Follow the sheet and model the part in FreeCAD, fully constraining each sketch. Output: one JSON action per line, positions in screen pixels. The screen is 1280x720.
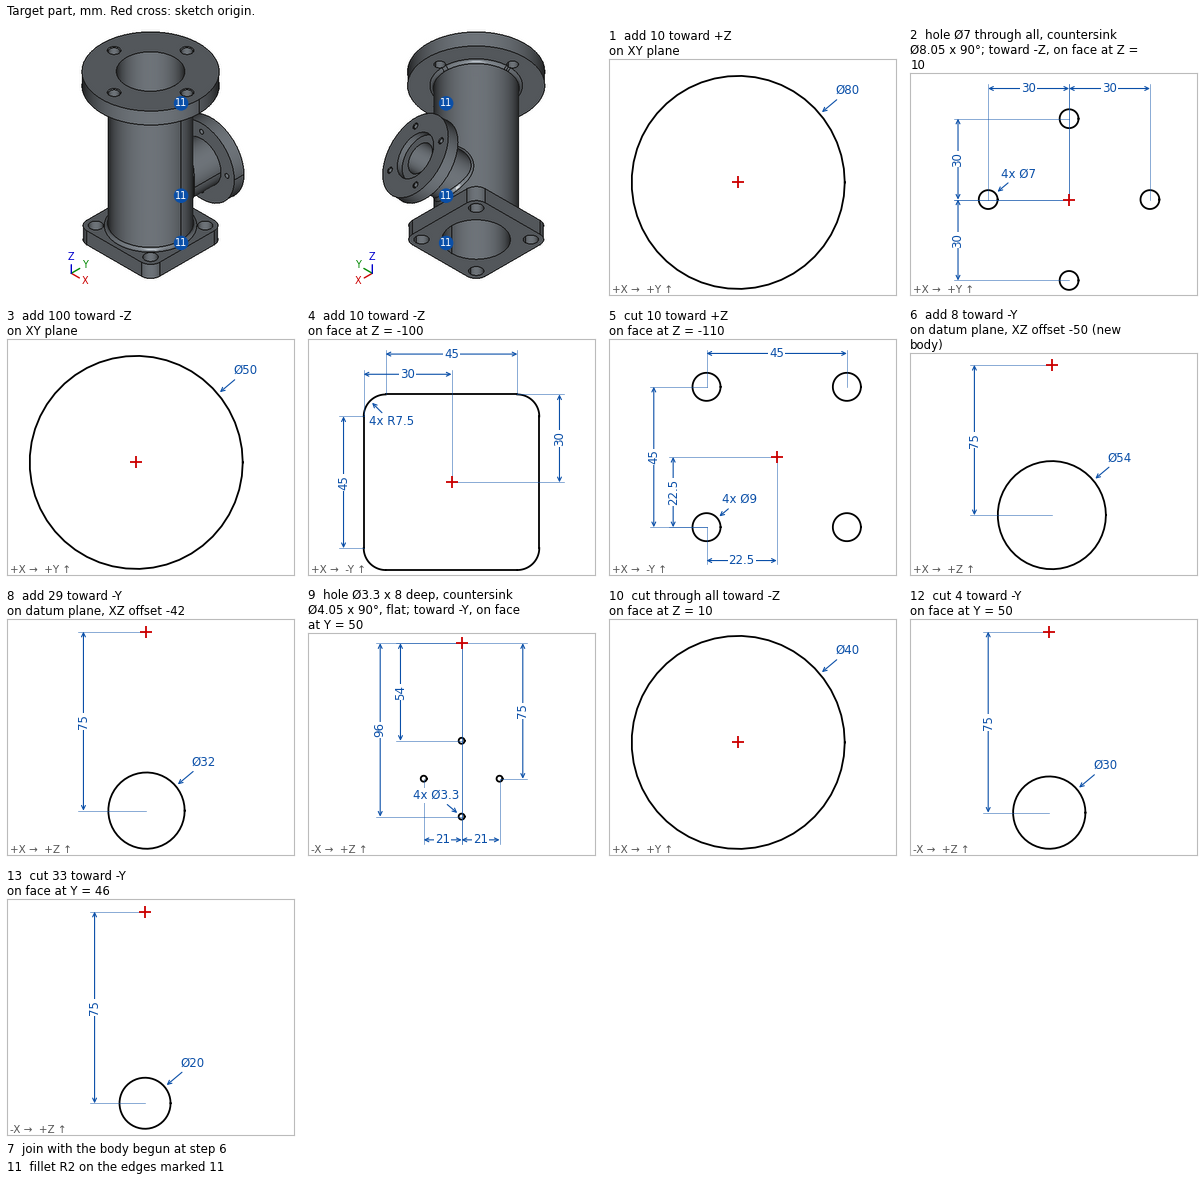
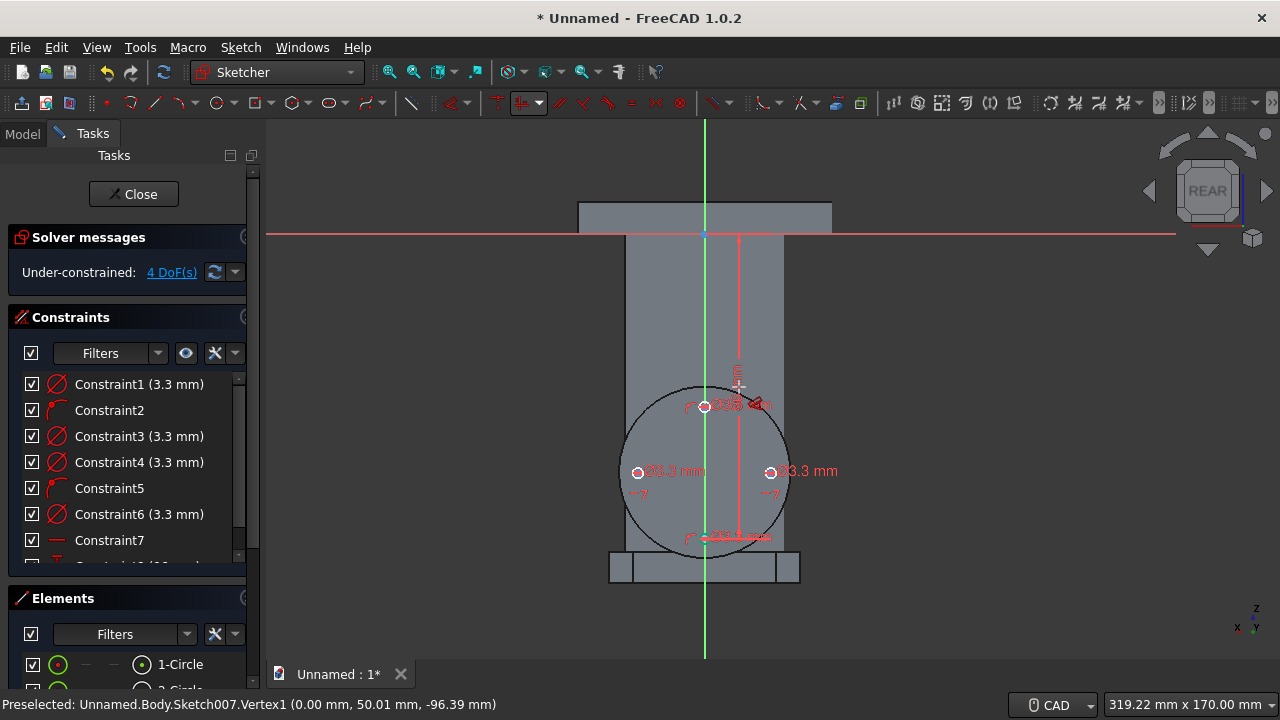
{"action": "left_click", "coordinate": [771, 473]}
{"action": "left_click", "coordinate": [738, 200]}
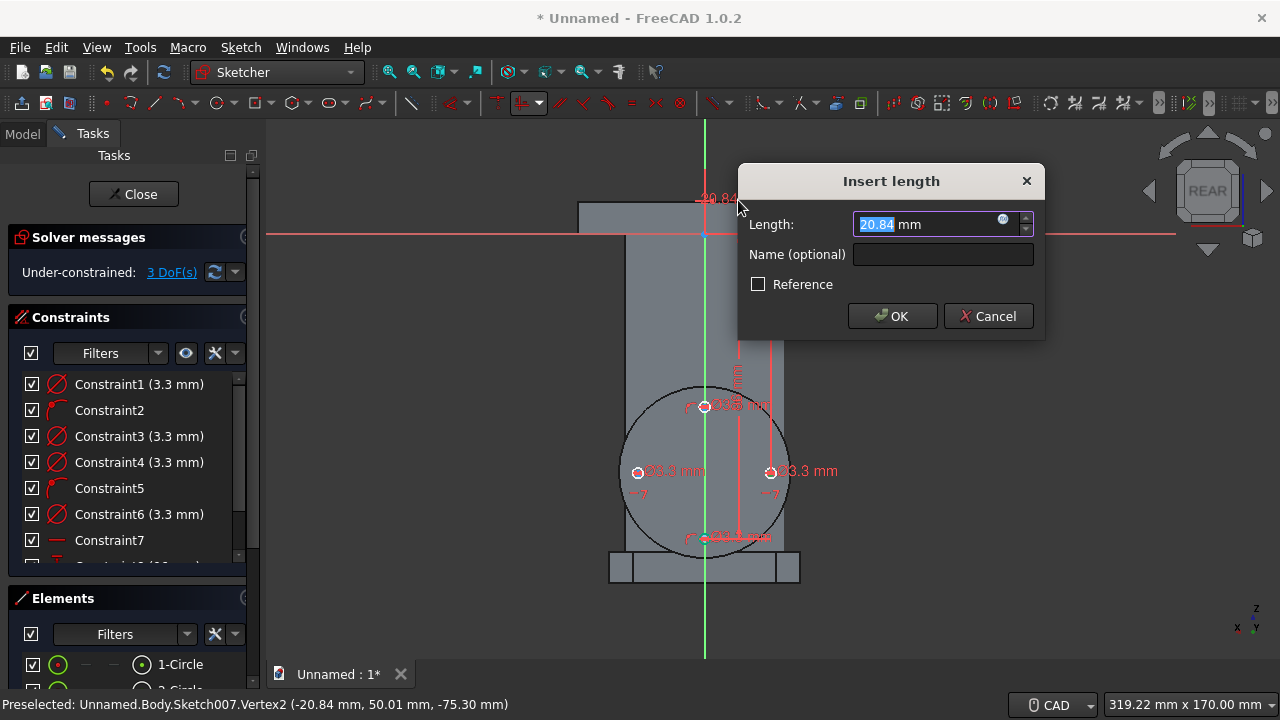
{"action": "type", "text": "21"}
{"action": "key", "text": "Return"}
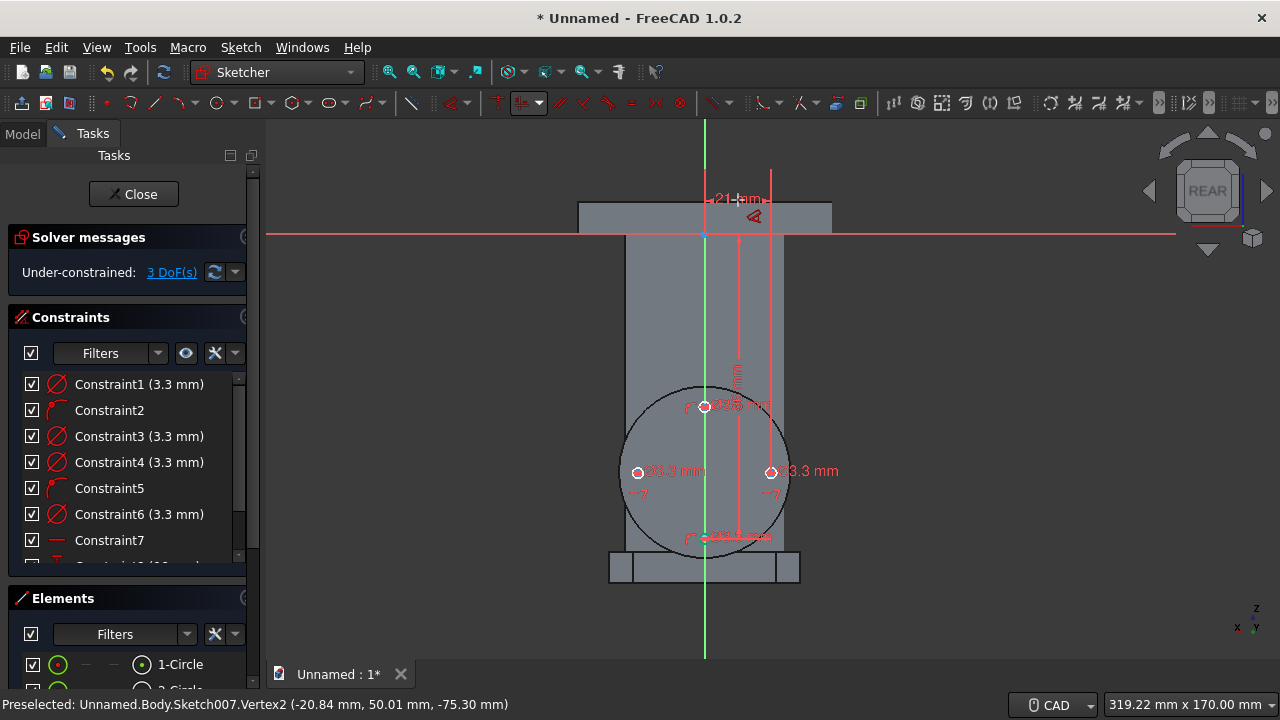
{"action": "left_click", "coordinate": [771, 473]}
{"action": "left_click", "coordinate": [805, 354]}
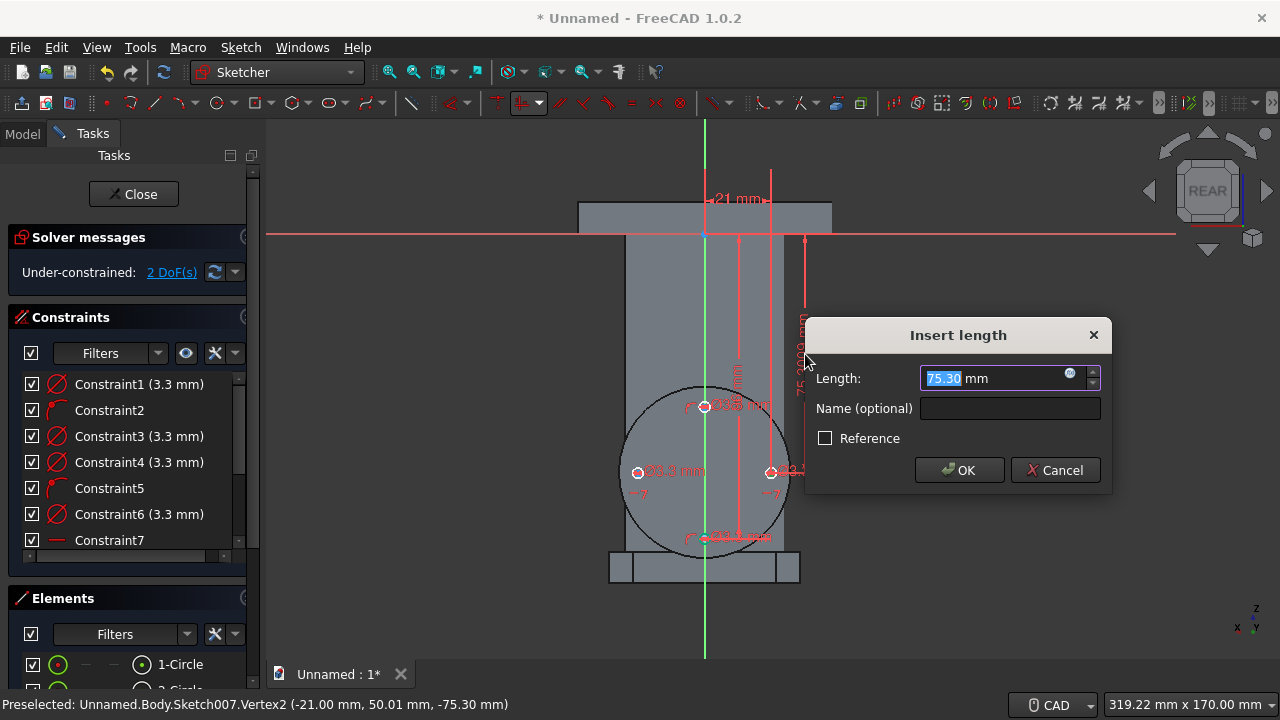
{"action": "type", "text": "75"}
{"action": "key", "text": "Return"}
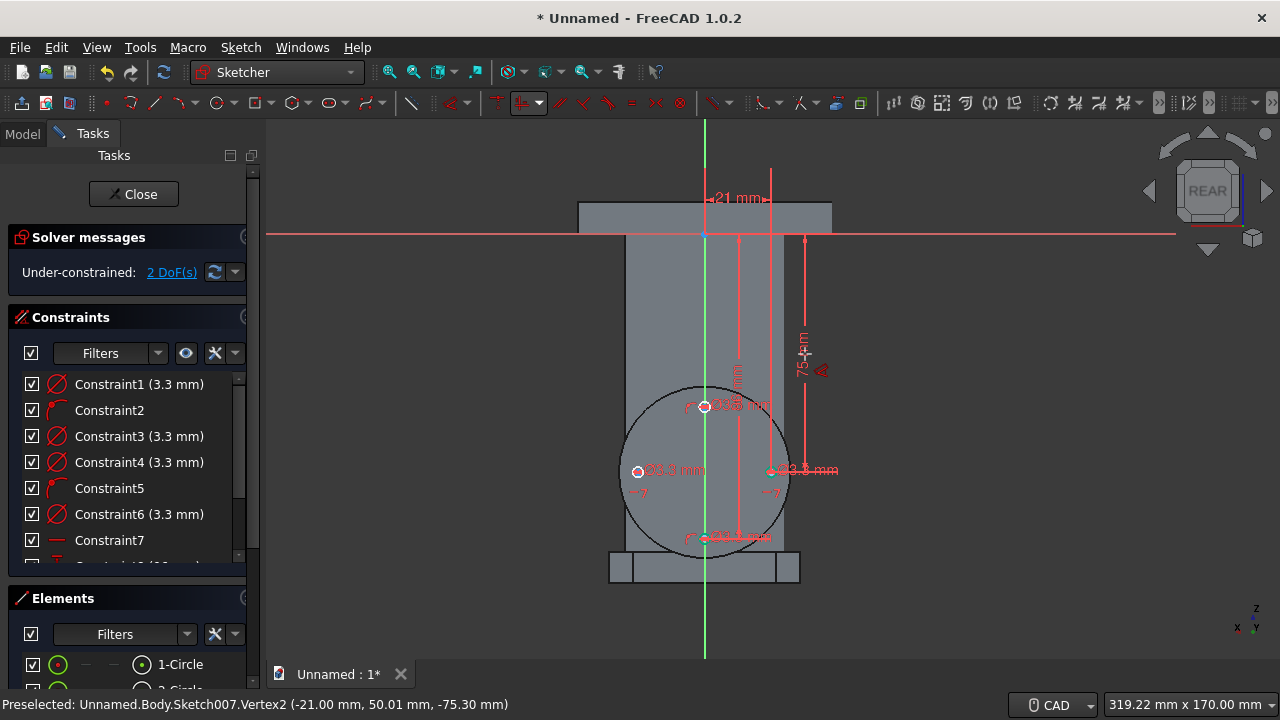
{"action": "left_click", "coordinate": [705, 407]}
{"action": "left_click", "coordinate": [739, 321]}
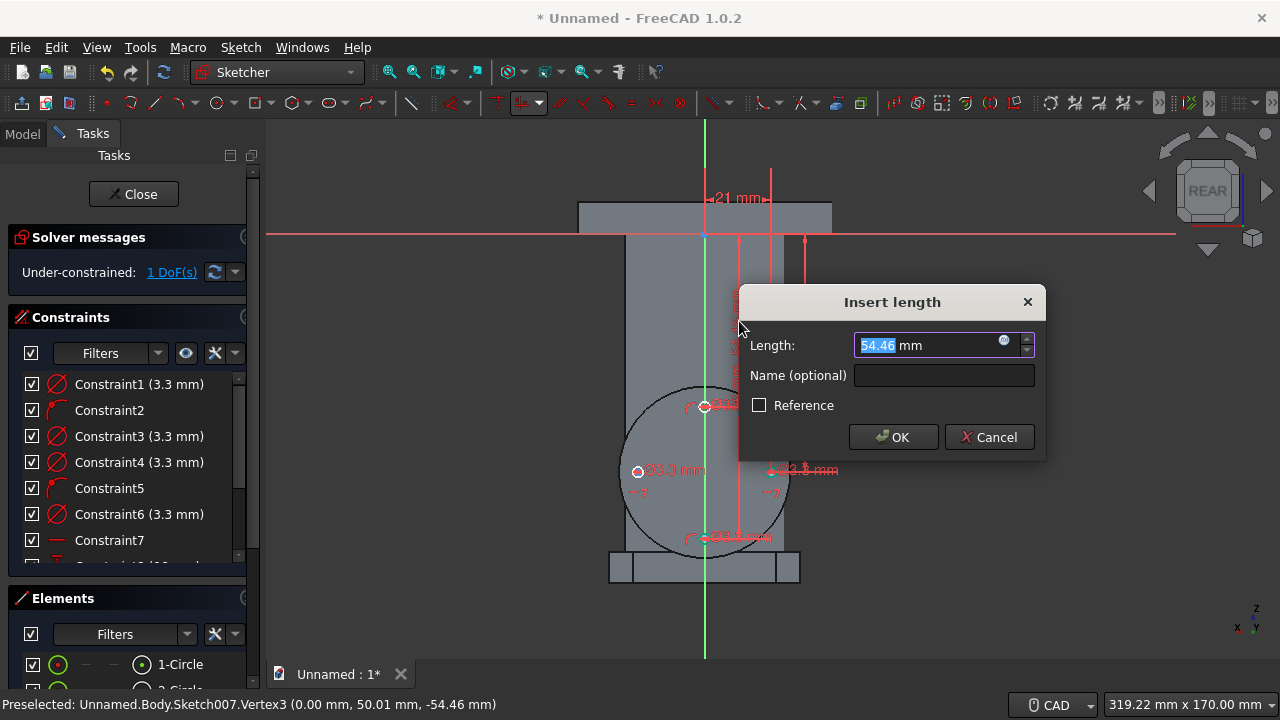
{"action": "type", "text": "54"}
{"action": "key", "text": "Return"}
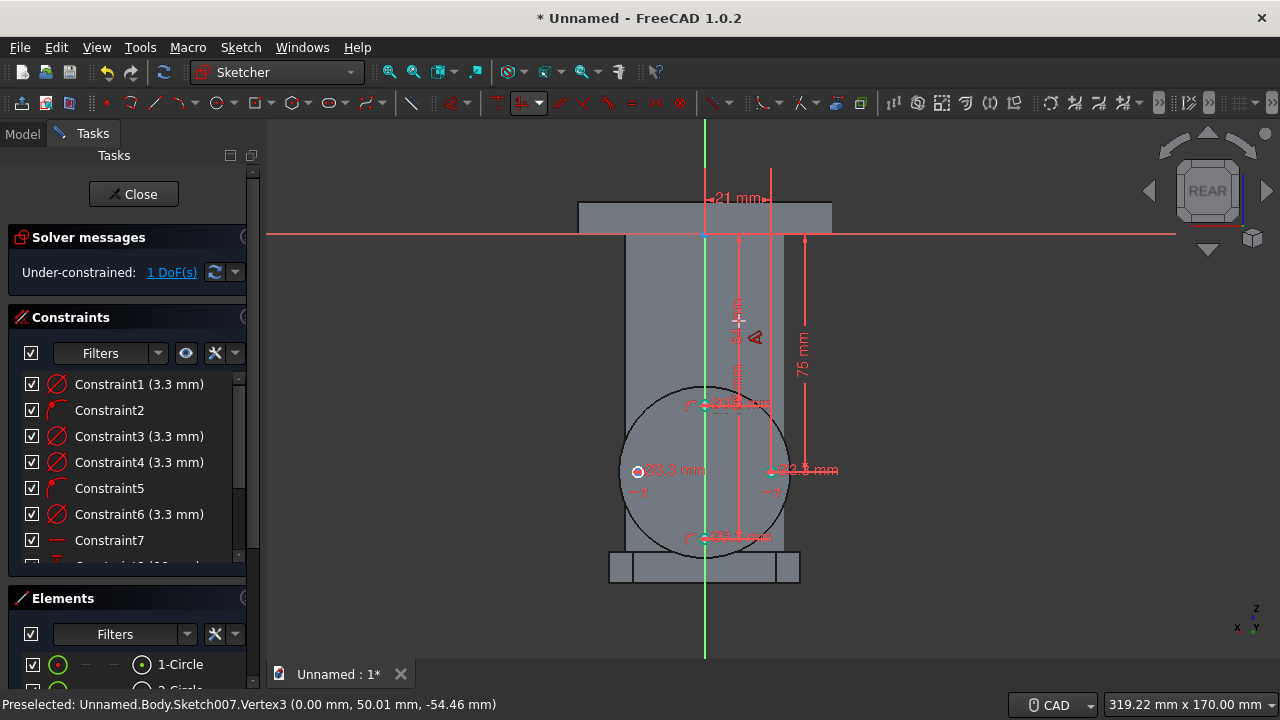
{"action": "left_click", "coordinate": [638, 472]}
{"action": "left_click", "coordinate": [656, 200]}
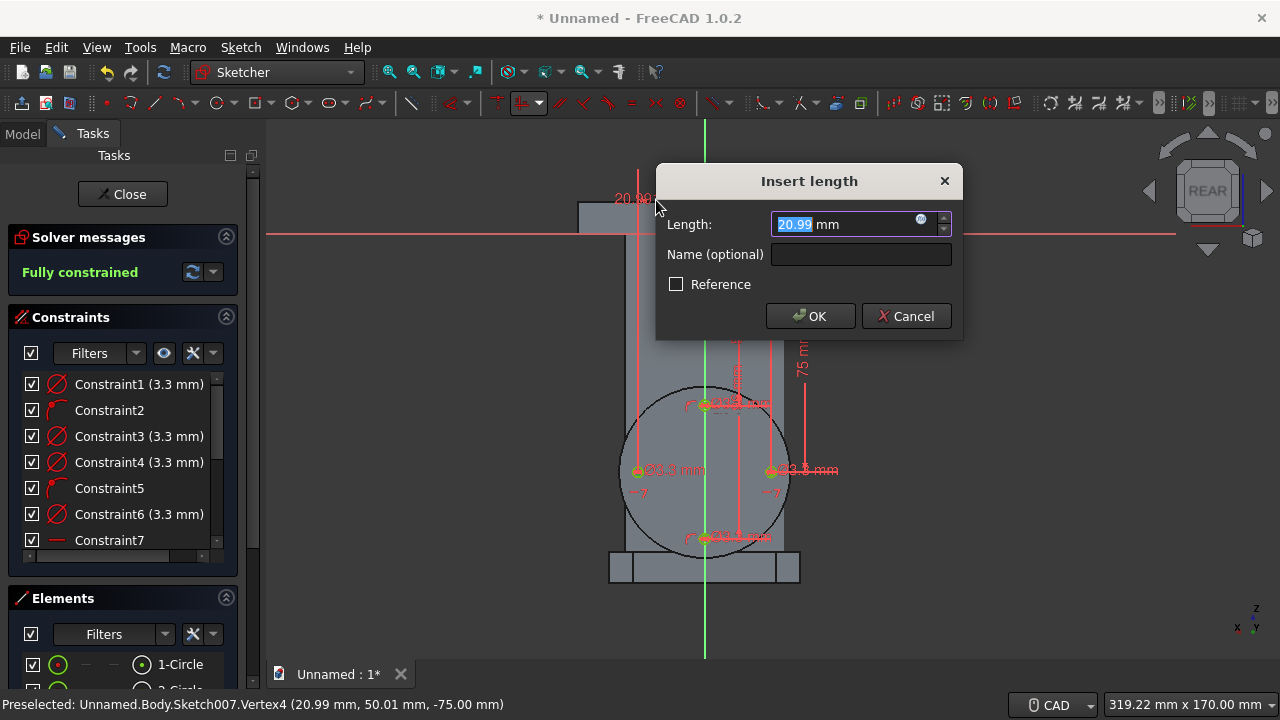
{"action": "type", "text": "21"}
{"action": "key", "text": "Return"}
{"action": "key", "text": "Escape"}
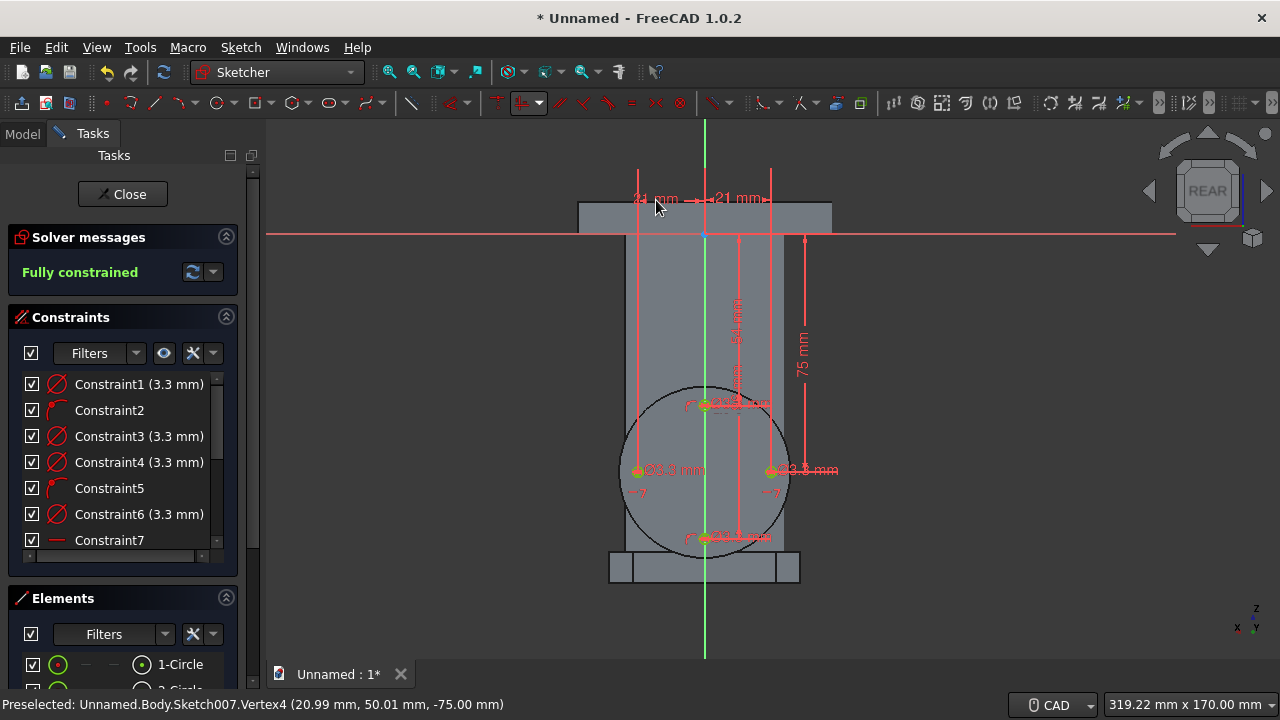
{"action": "left_click", "coordinate": [123, 194]}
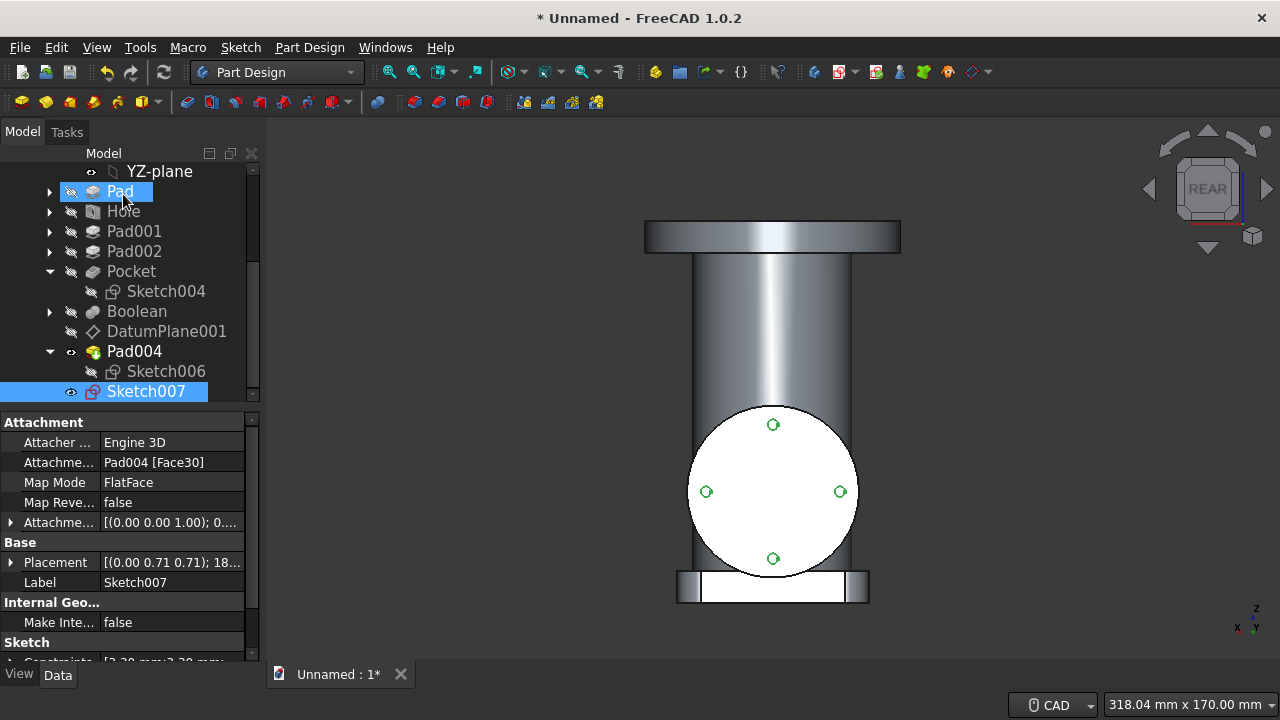
{"action": "left_click", "coordinate": [212, 102]}